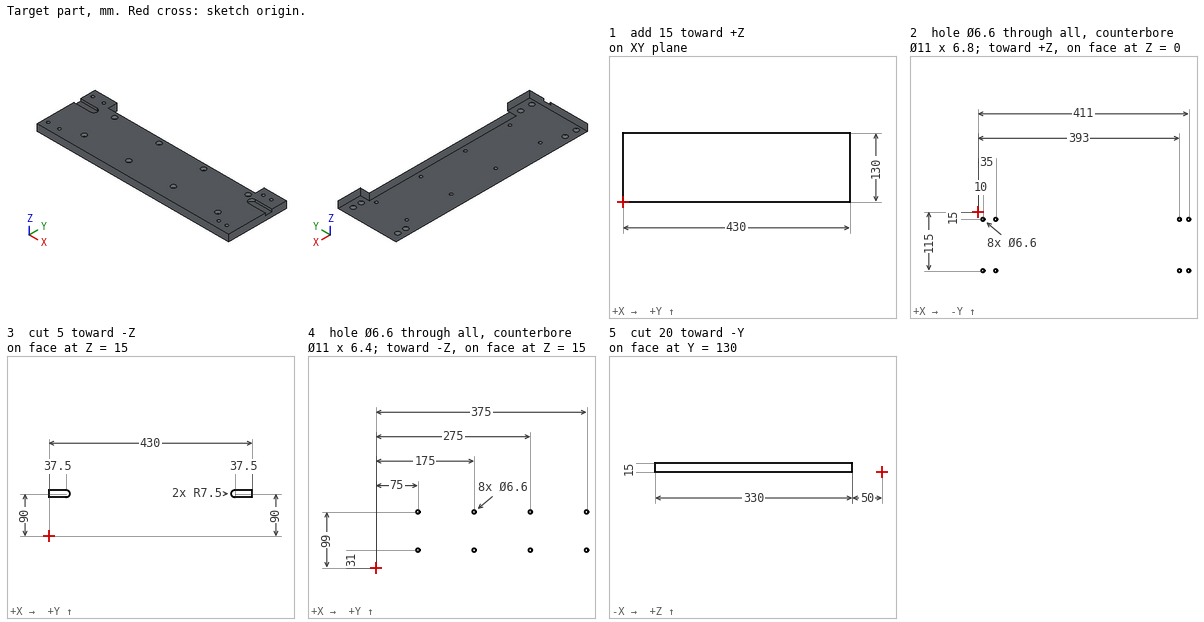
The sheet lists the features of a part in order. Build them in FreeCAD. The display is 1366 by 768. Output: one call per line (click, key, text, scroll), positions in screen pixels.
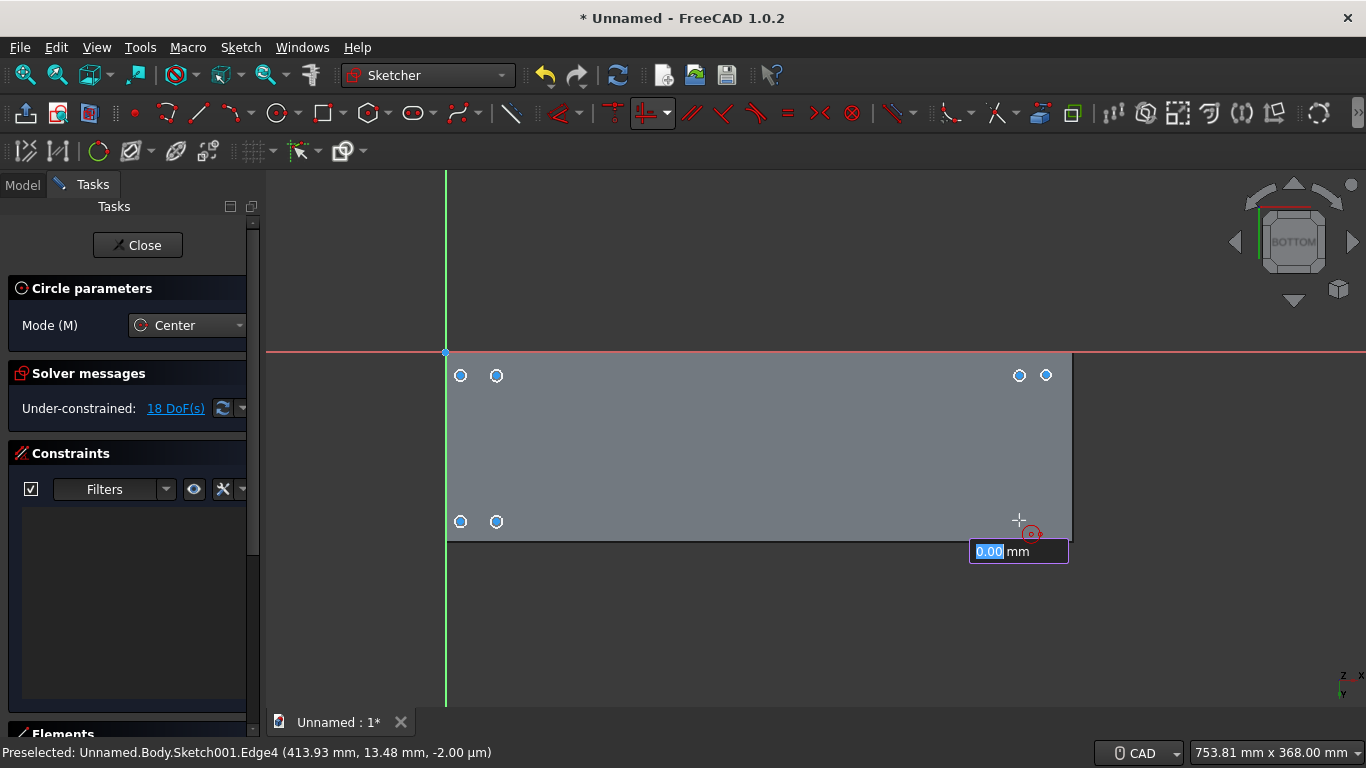
scroll(1023, 517, up, 6)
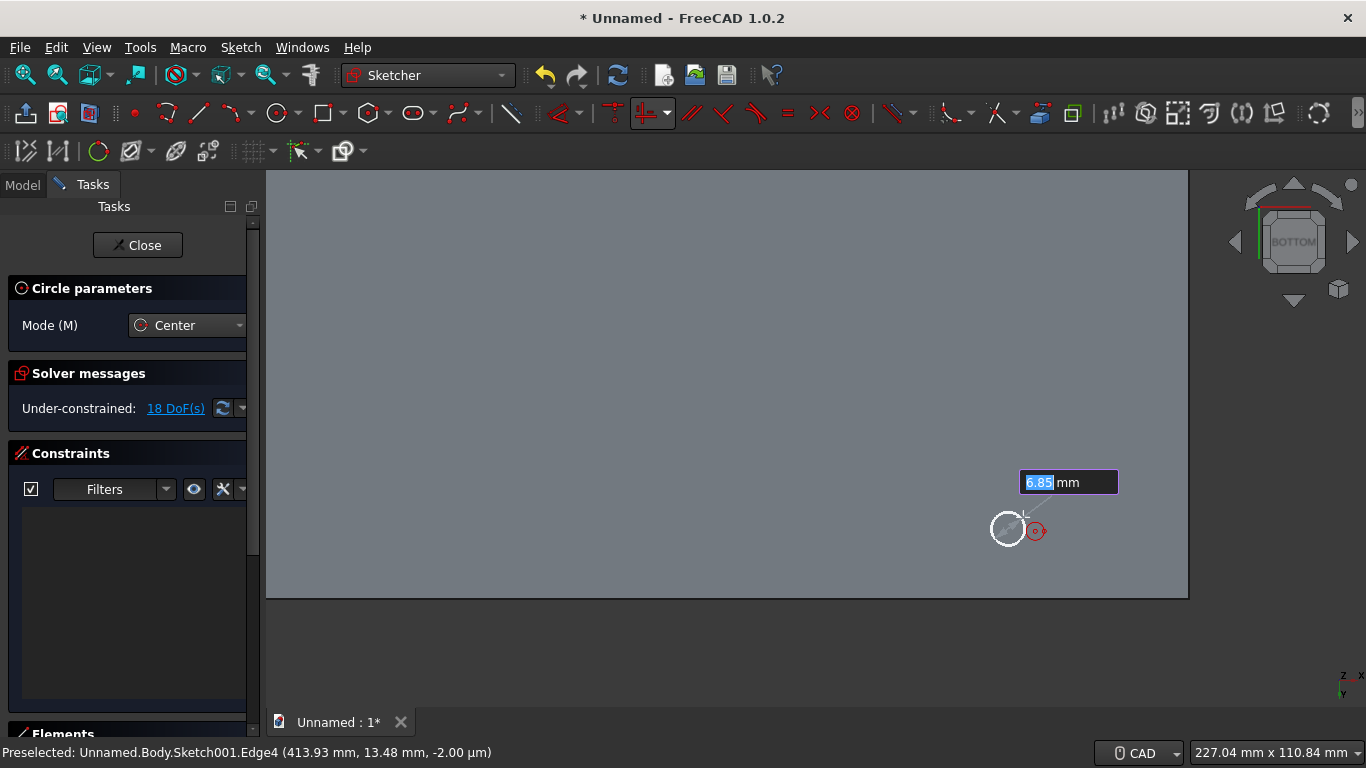
click(1021, 515)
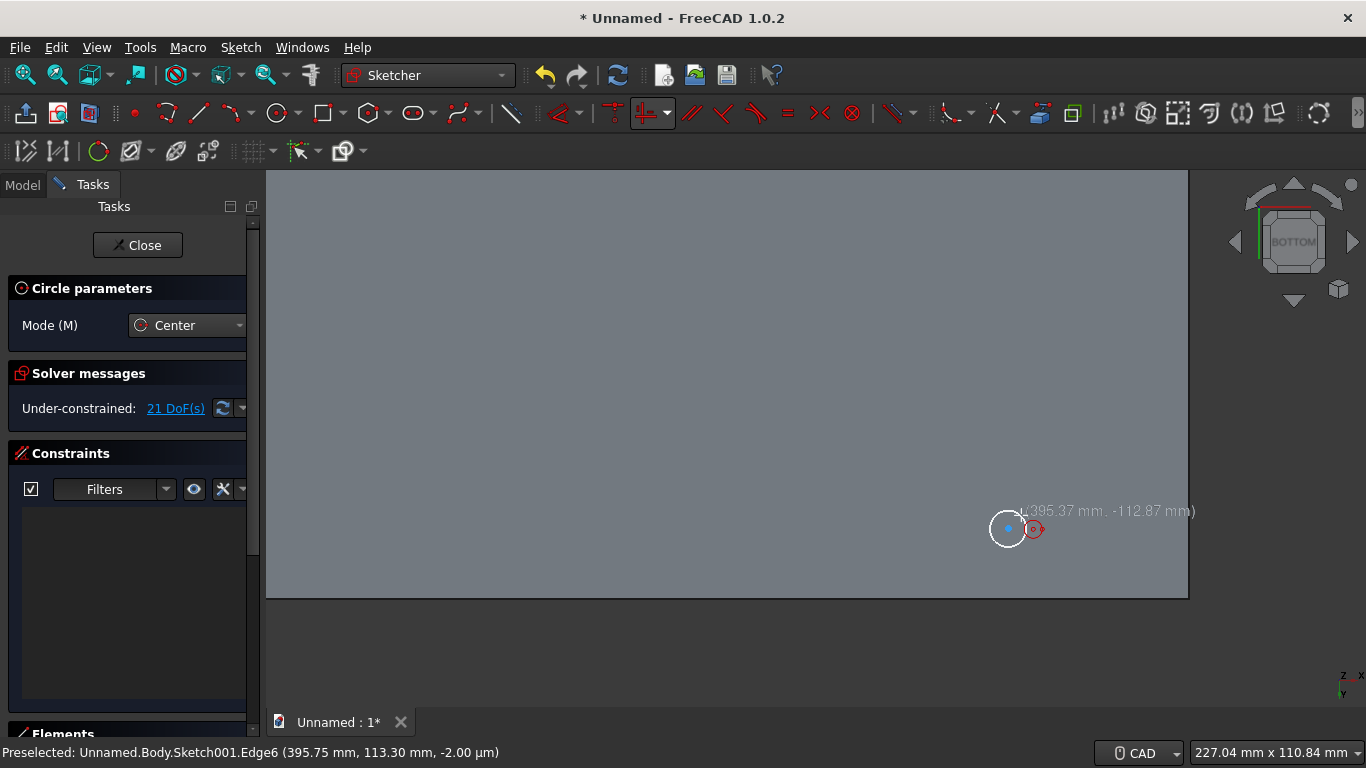
scroll(1097, 526, up, 2)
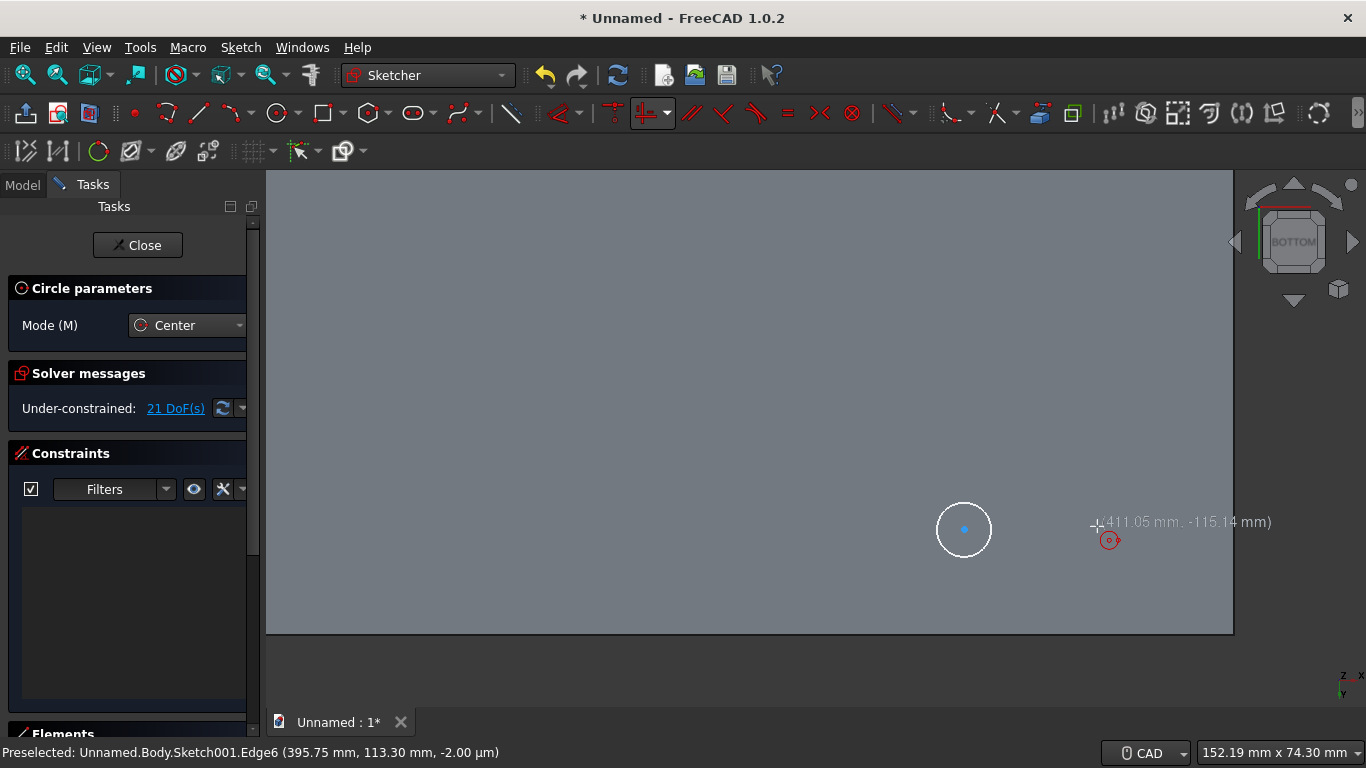
scroll(1032, 518, down, 8)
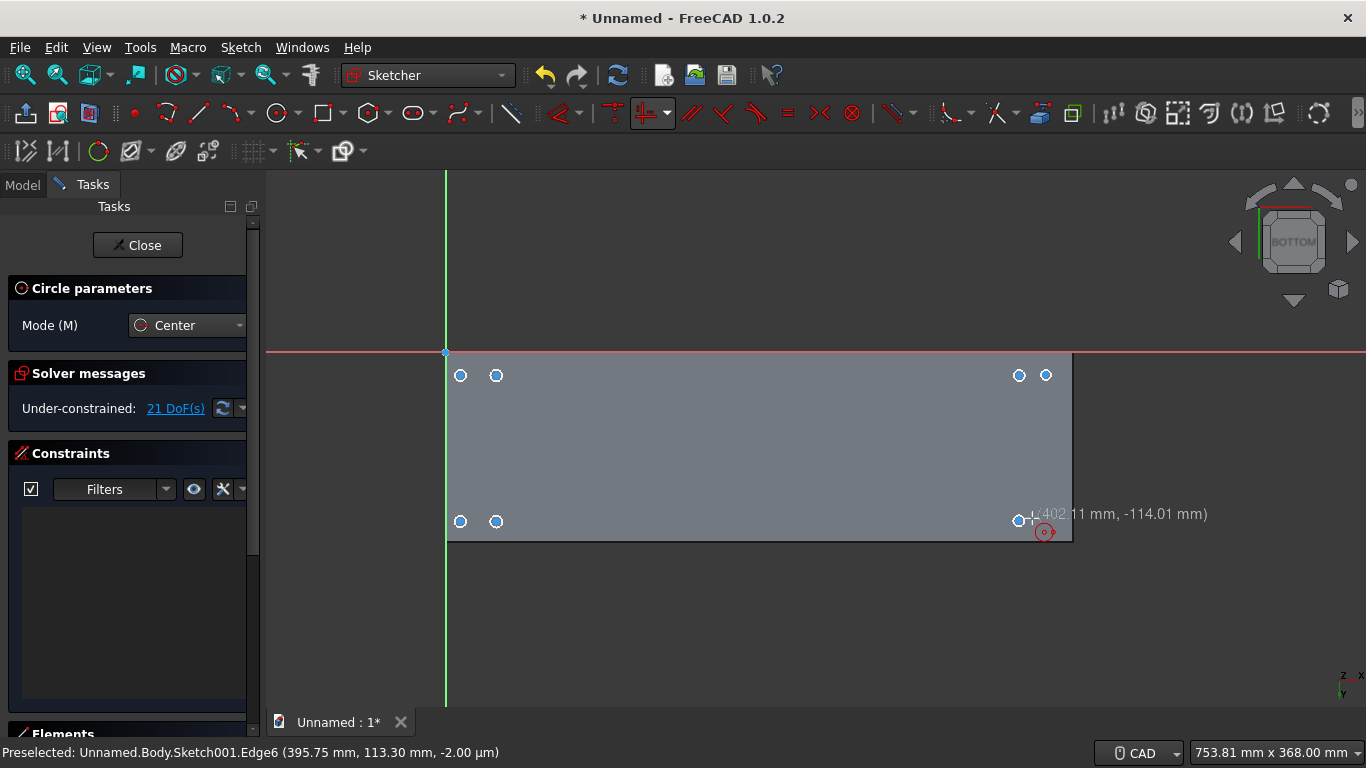
click(1046, 520)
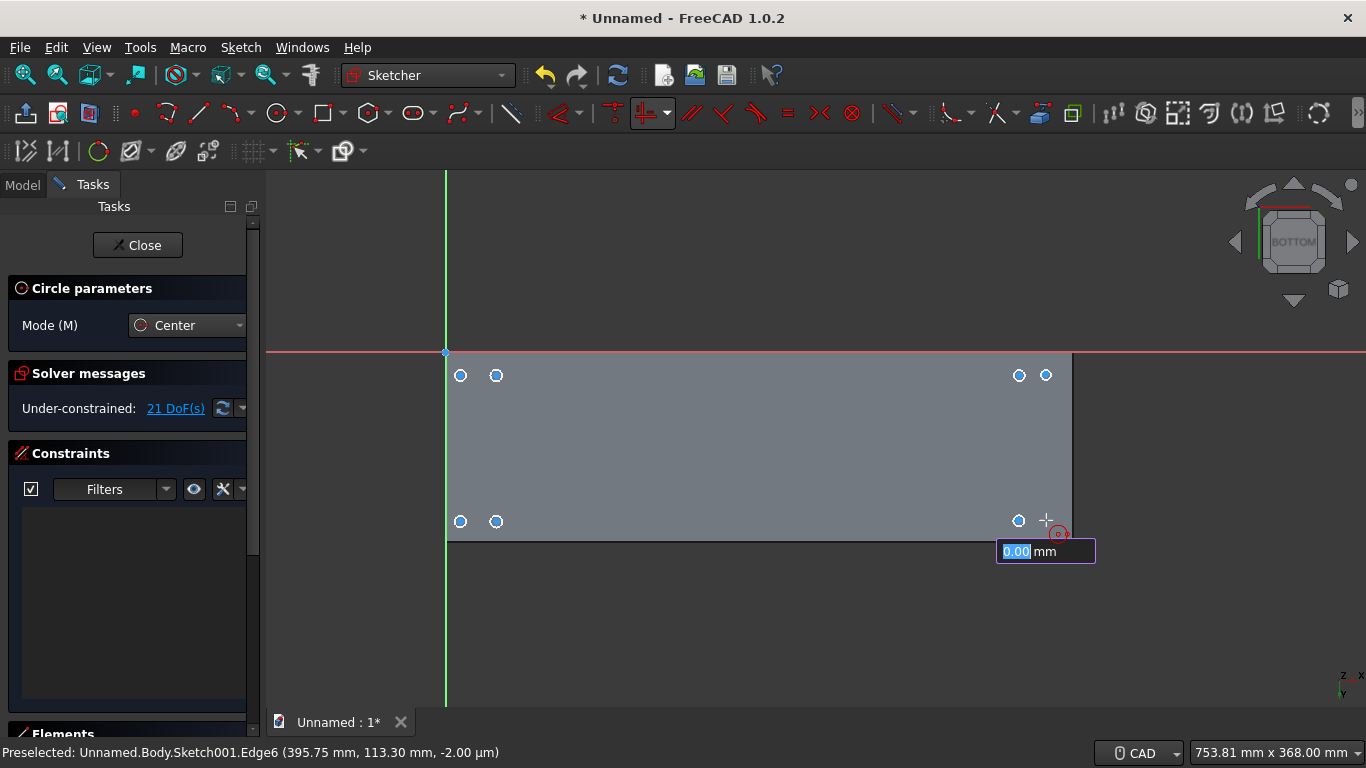
scroll(1049, 517, up, 6)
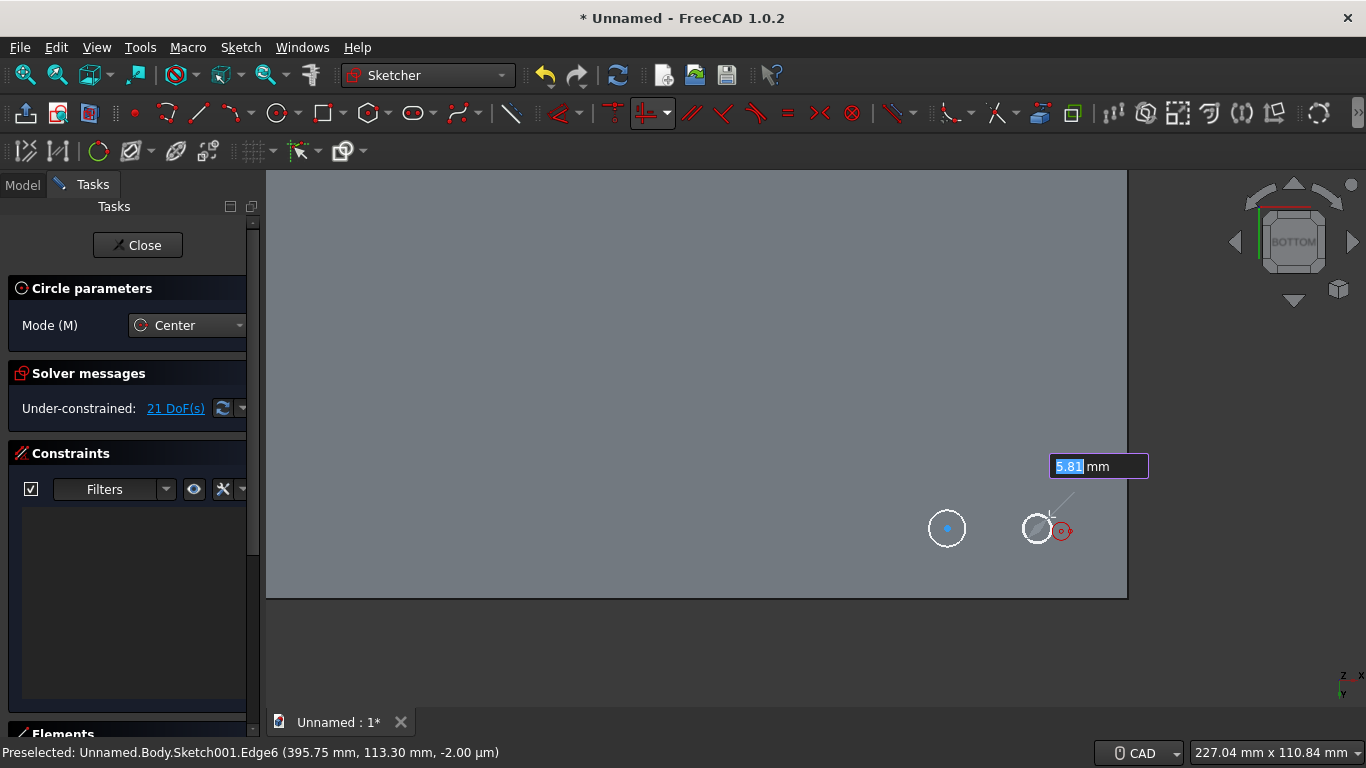
click(1047, 515)
key(Escape)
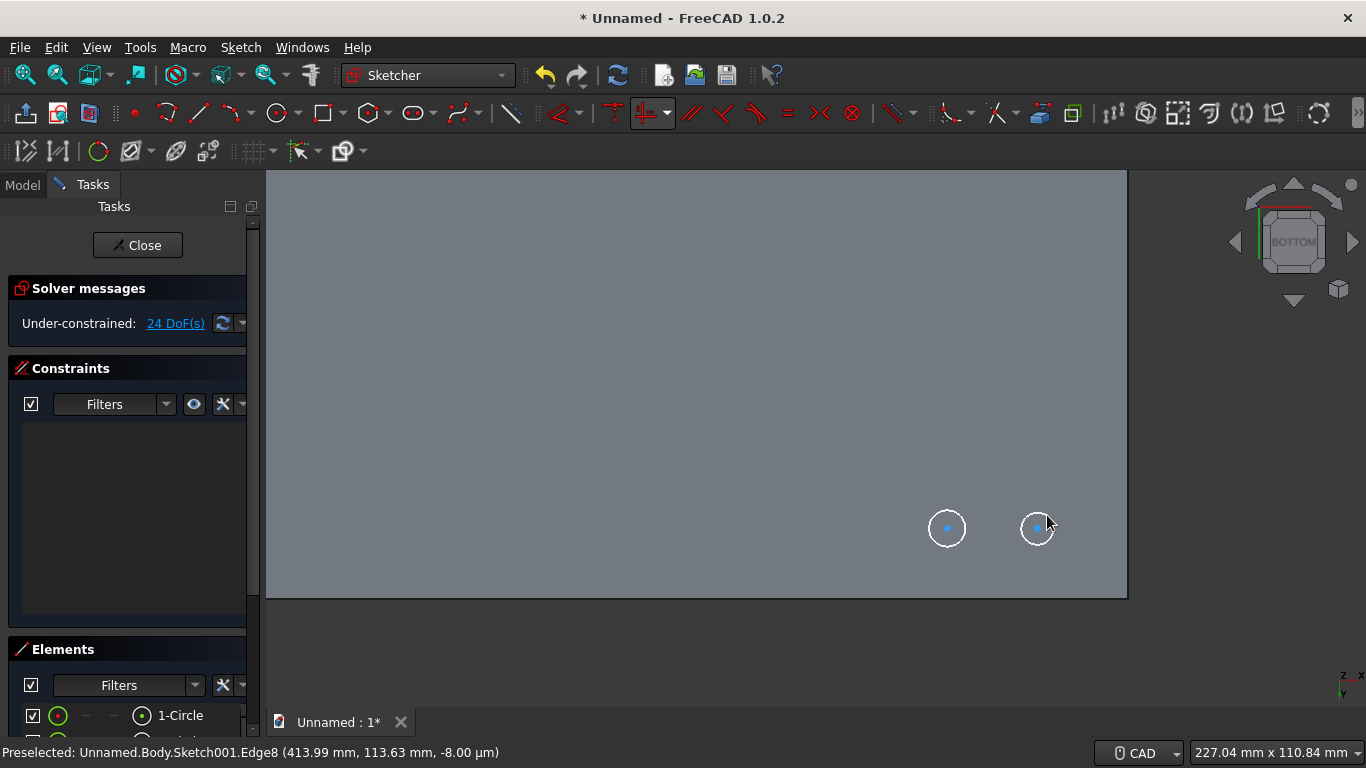
scroll(1049, 517, down, 6)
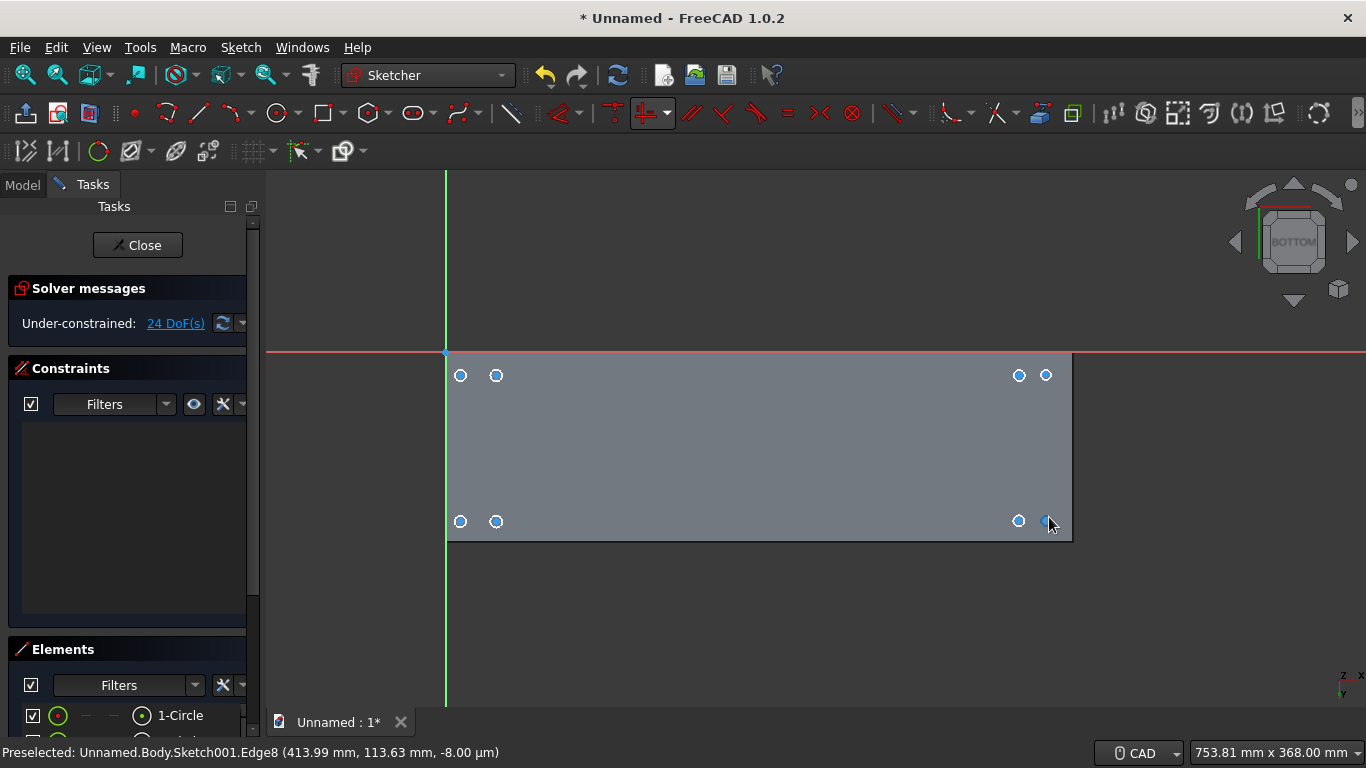
scroll(464, 372, up, 5)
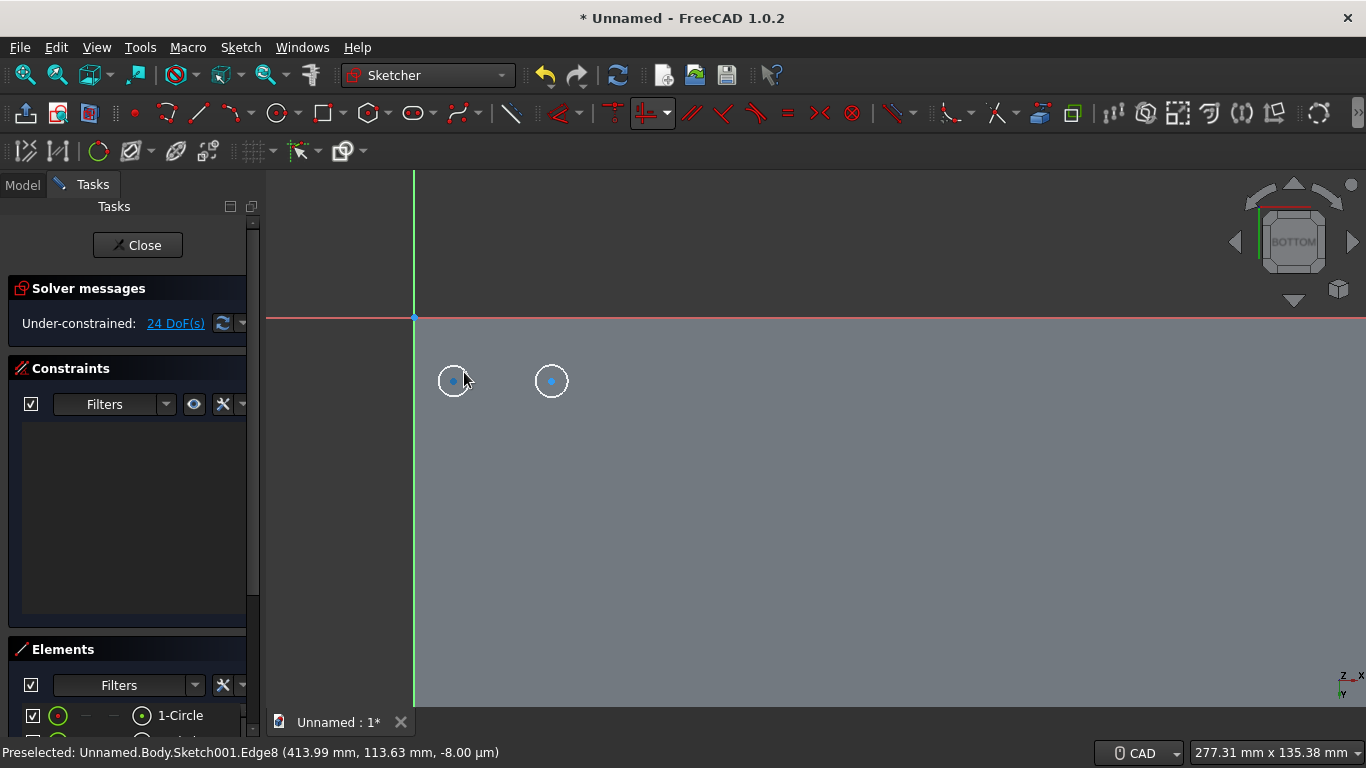
click(465, 370)